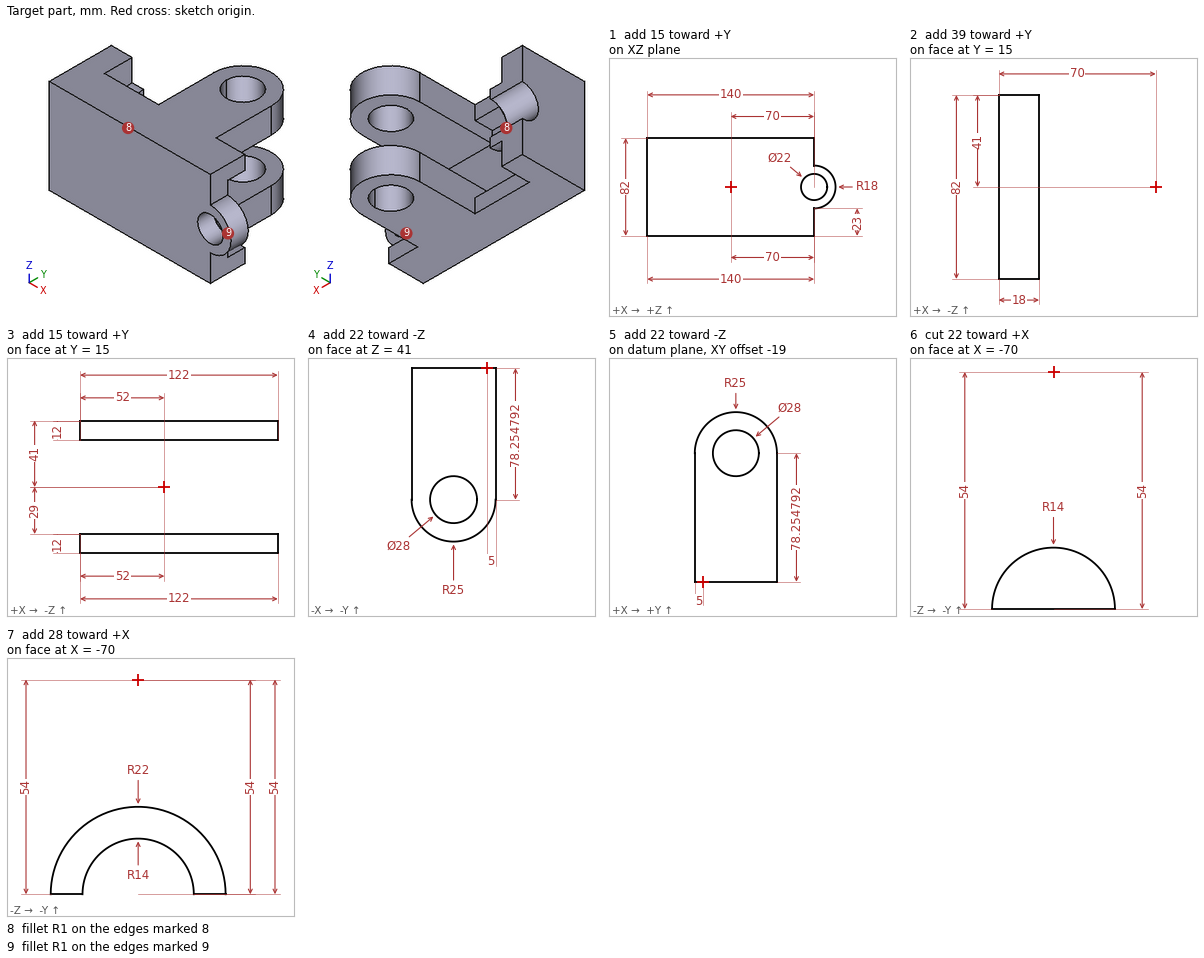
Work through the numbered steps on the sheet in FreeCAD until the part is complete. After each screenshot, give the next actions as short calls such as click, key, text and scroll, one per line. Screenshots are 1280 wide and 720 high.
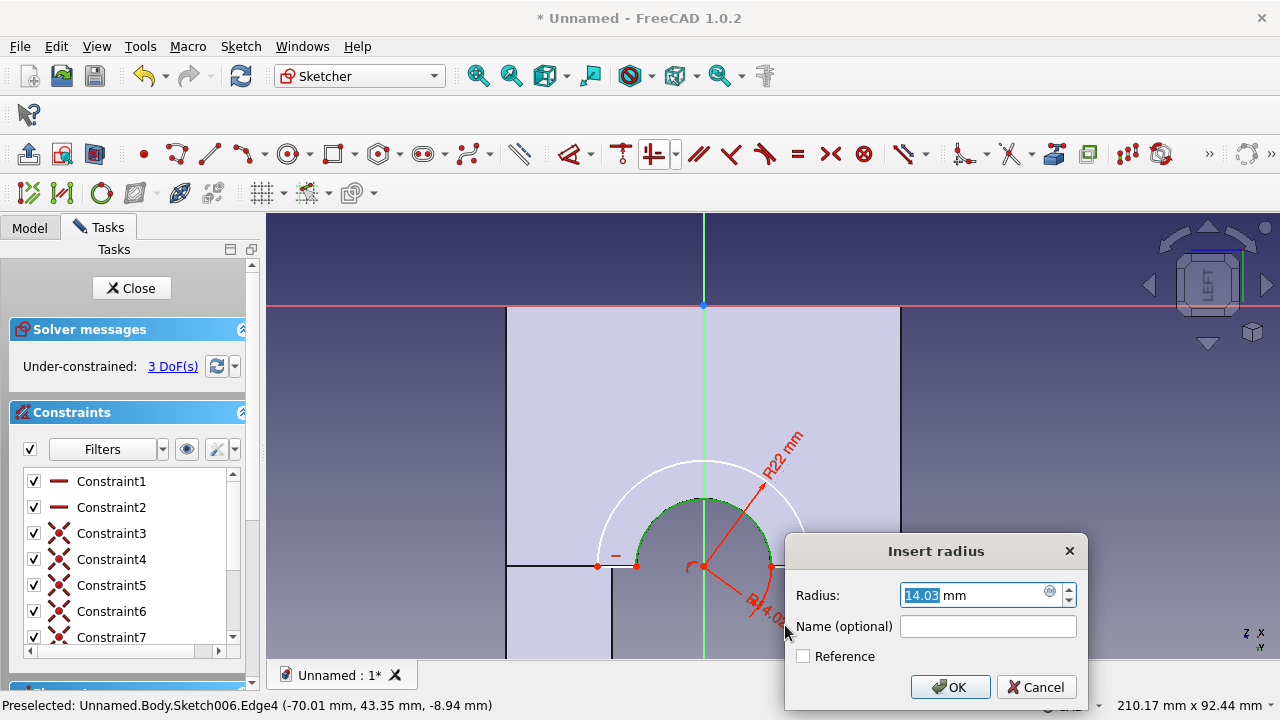
text(14)
key(Return)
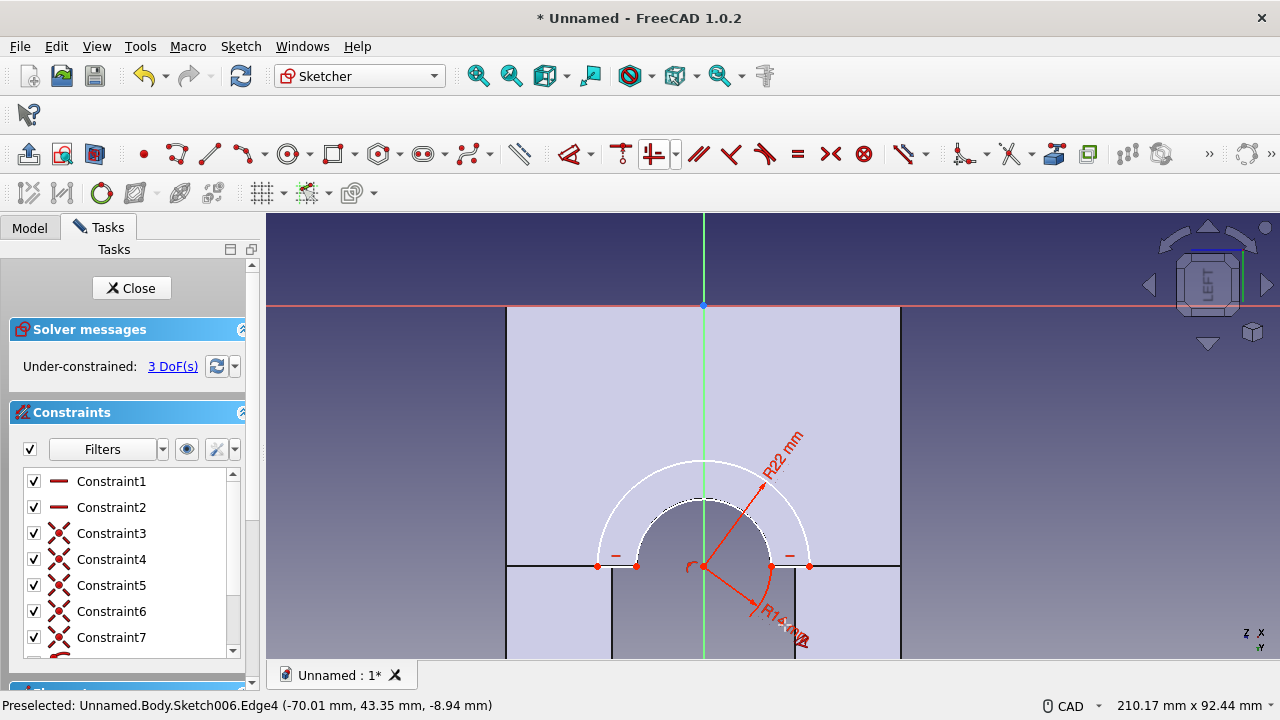
click(771, 567)
click(805, 376)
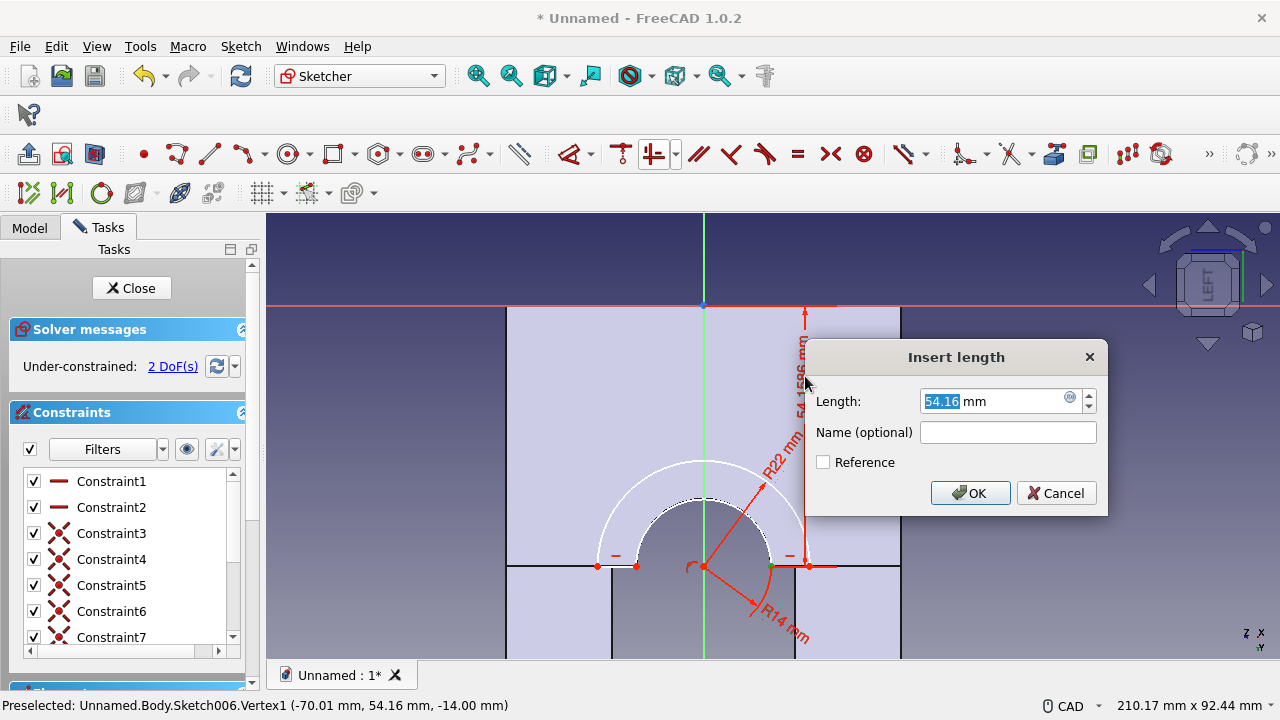
text(54)
key(Return)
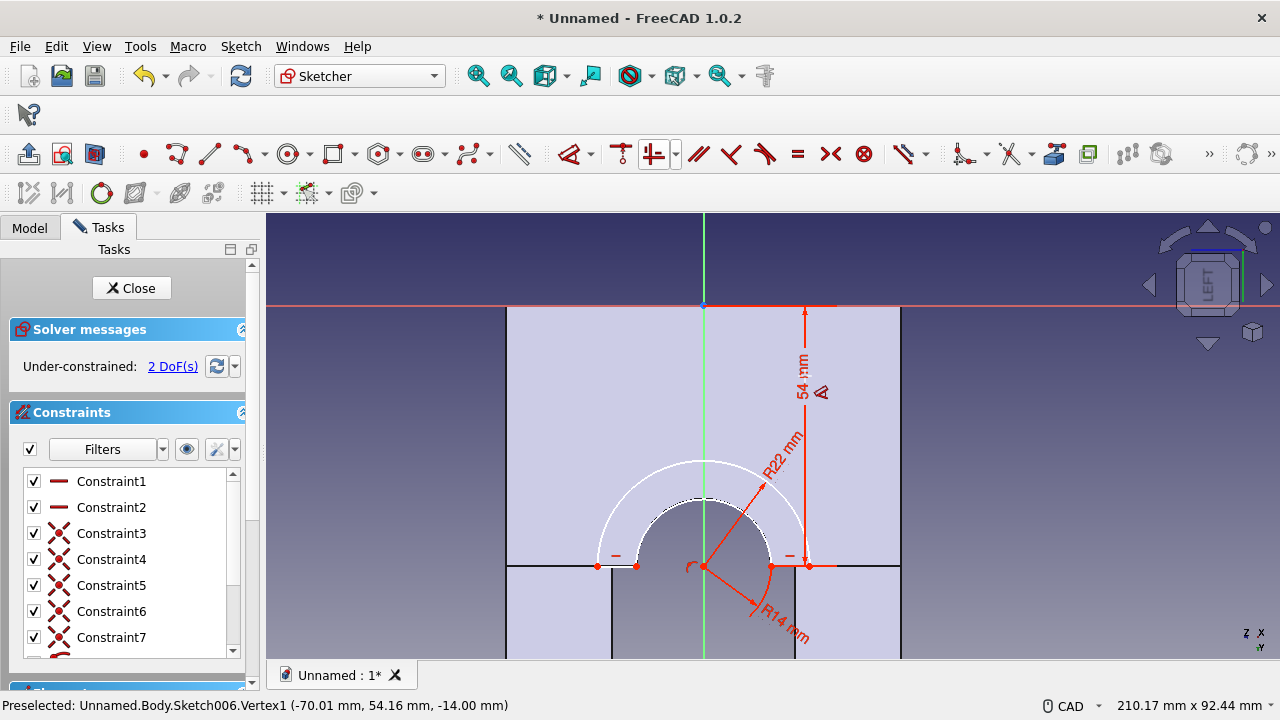
click(598, 567)
click(564, 436)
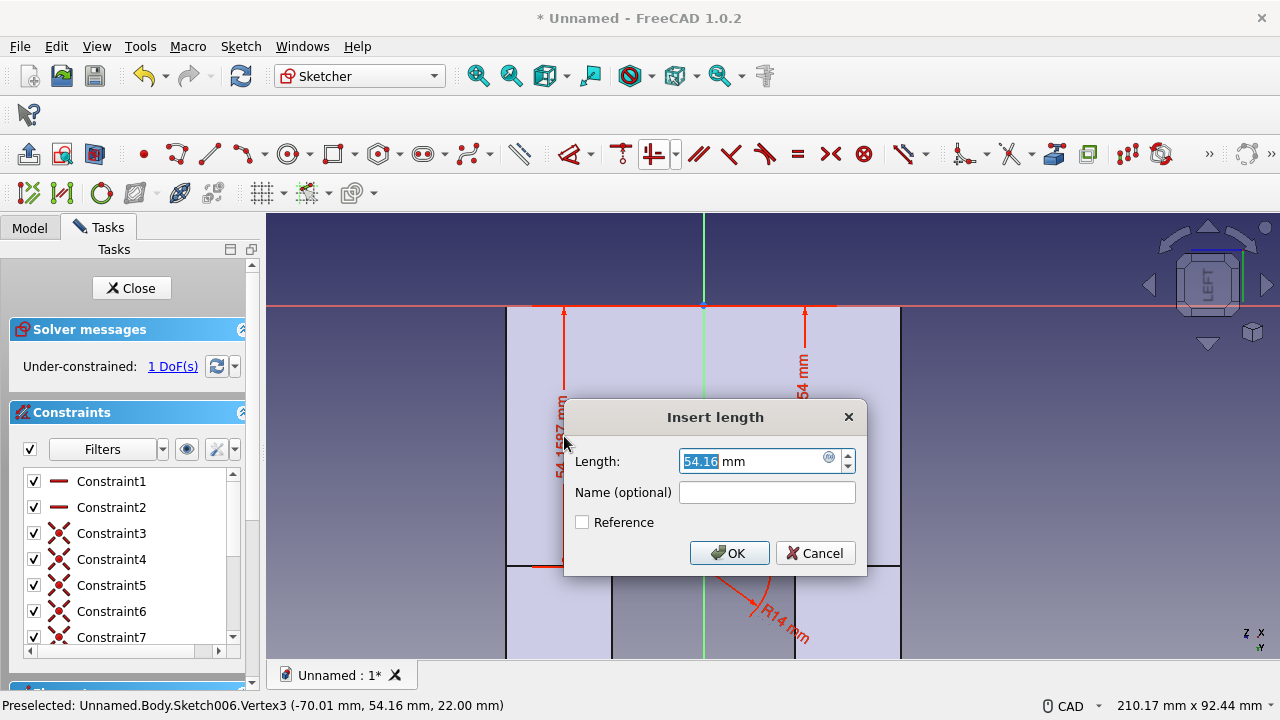
text(54)
key(Return)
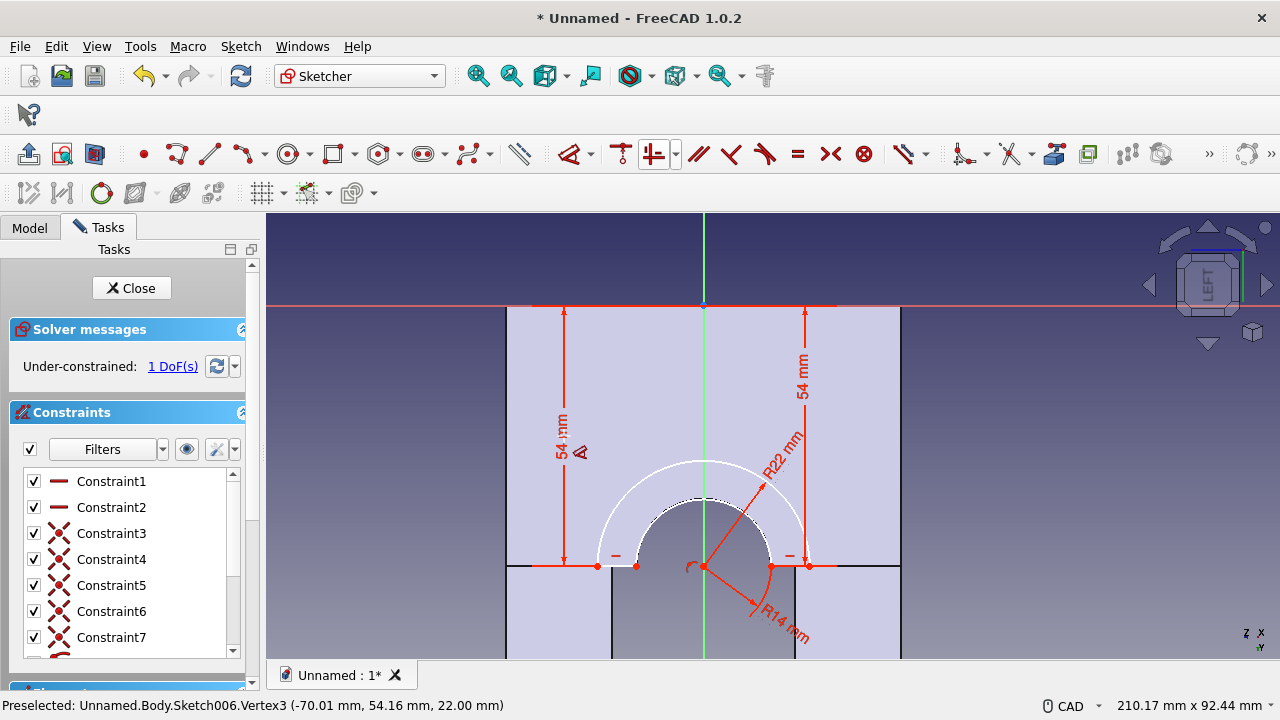
click(704, 567)
click(738, 345)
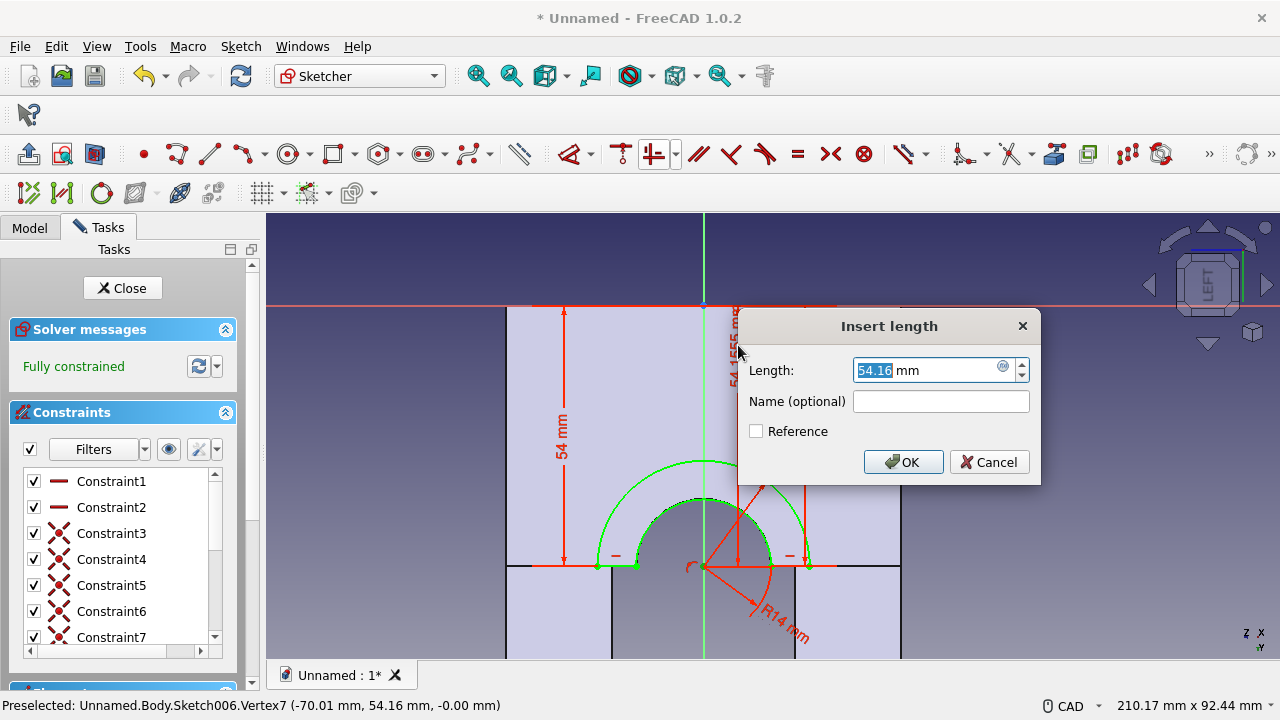
text(54)
key(Return)
key(Escape)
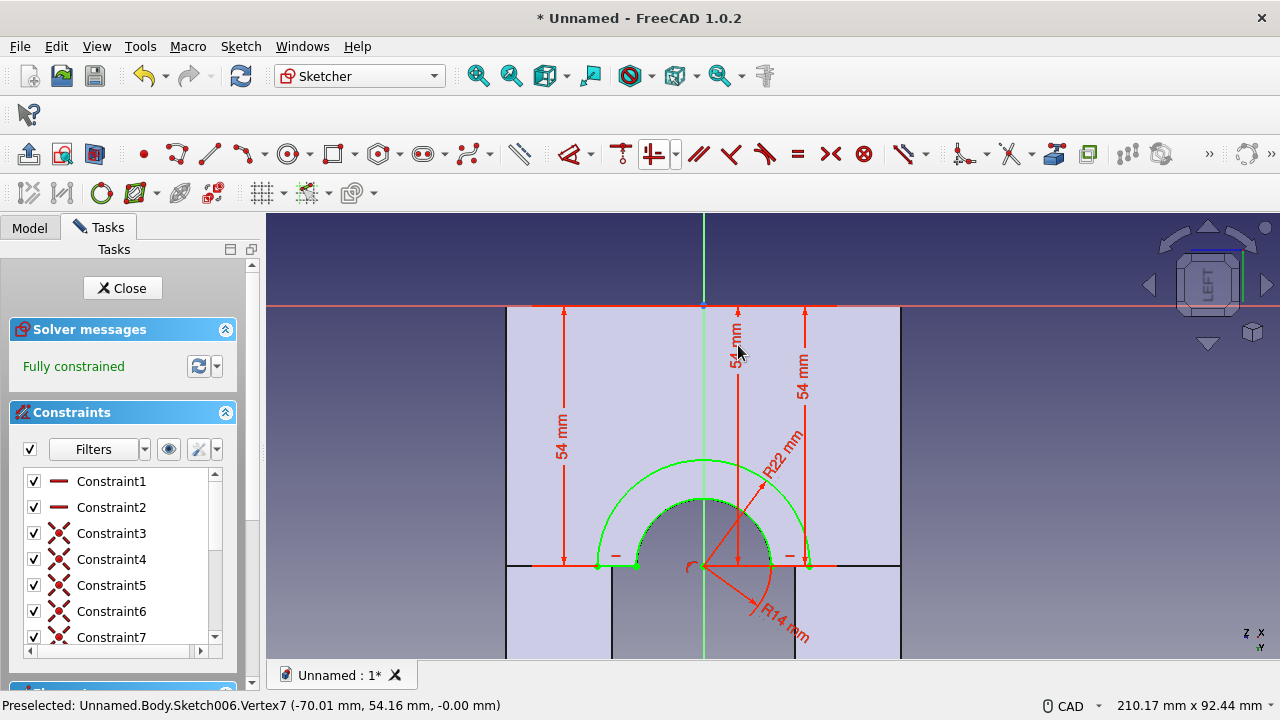
click(123, 288)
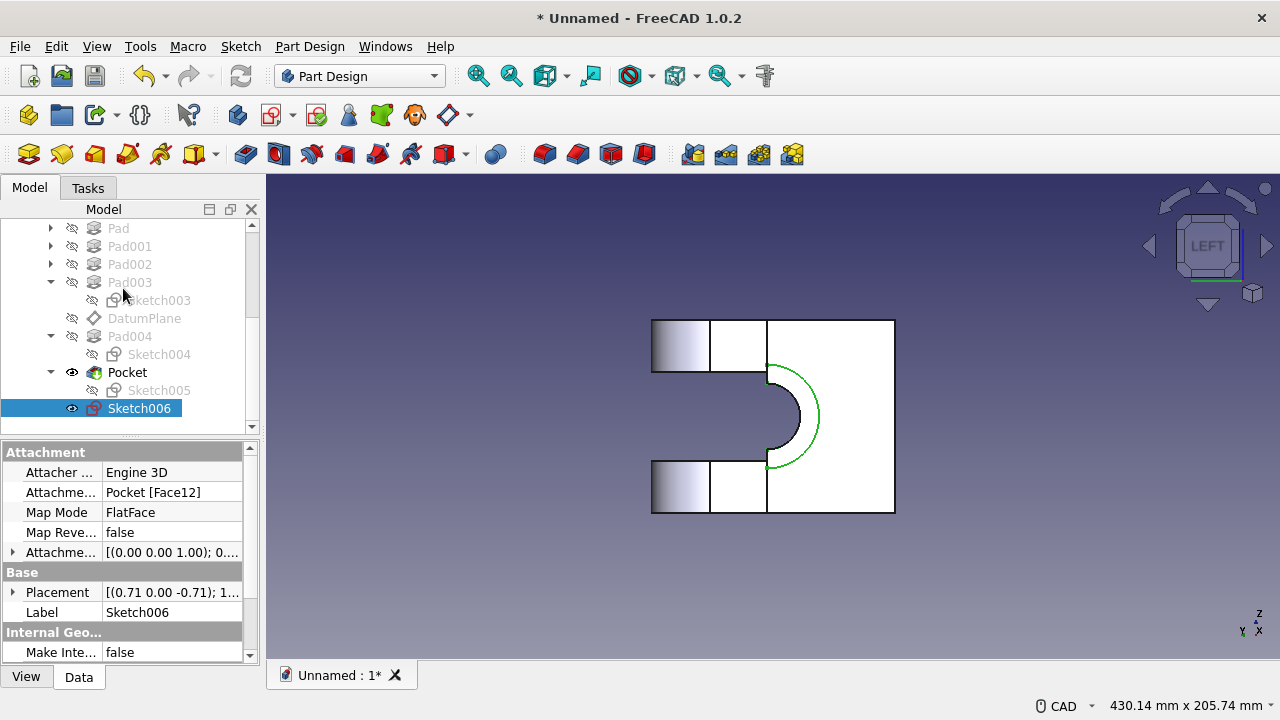
click(29, 154)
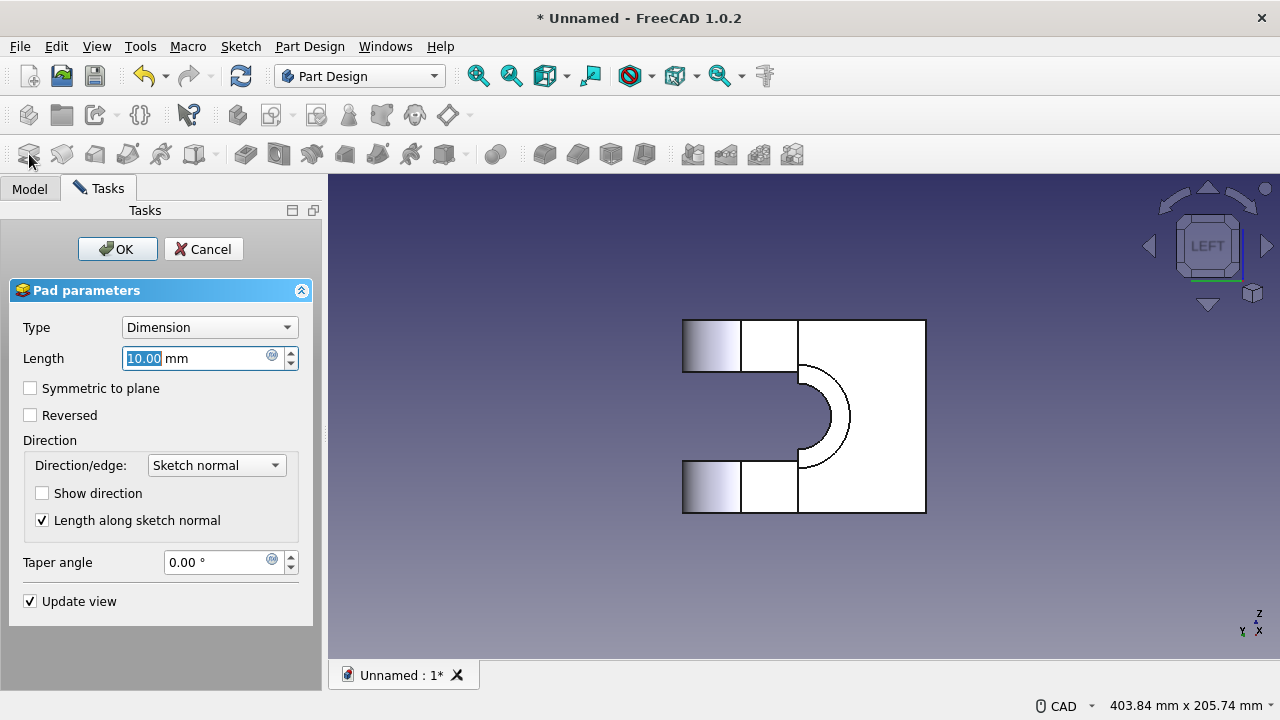
text(28)
key(Tab)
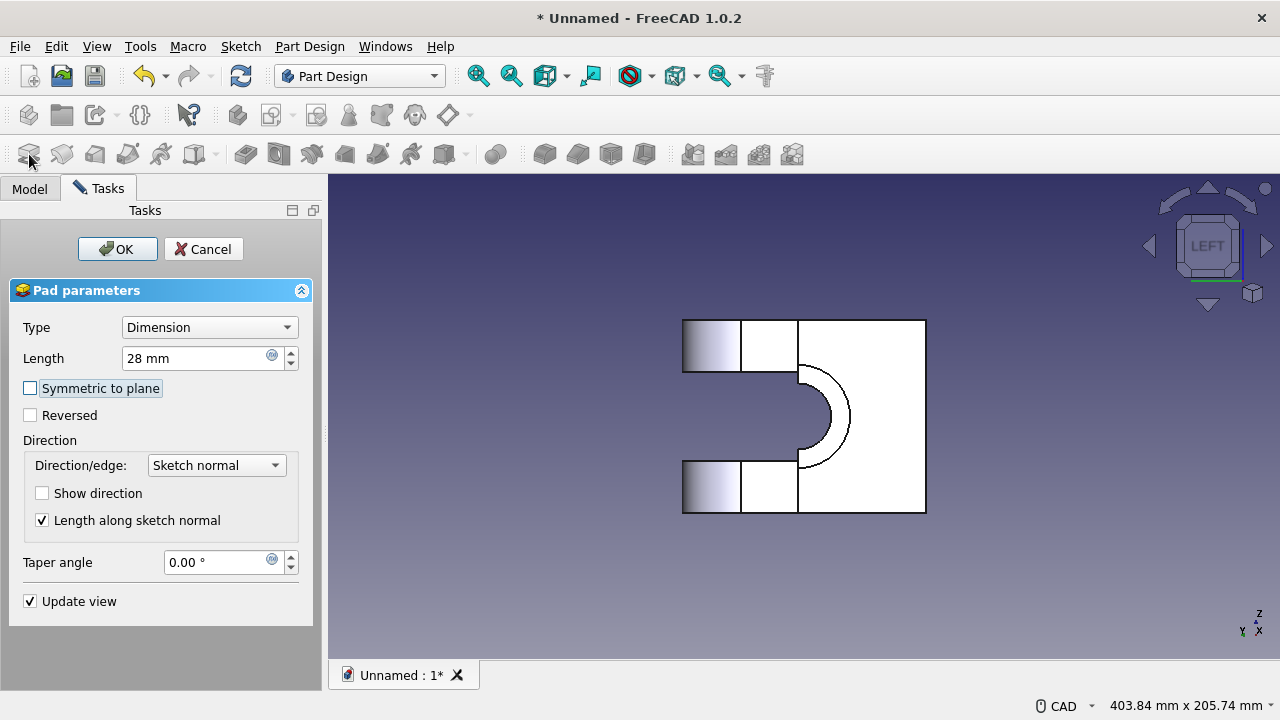
click(31, 415)